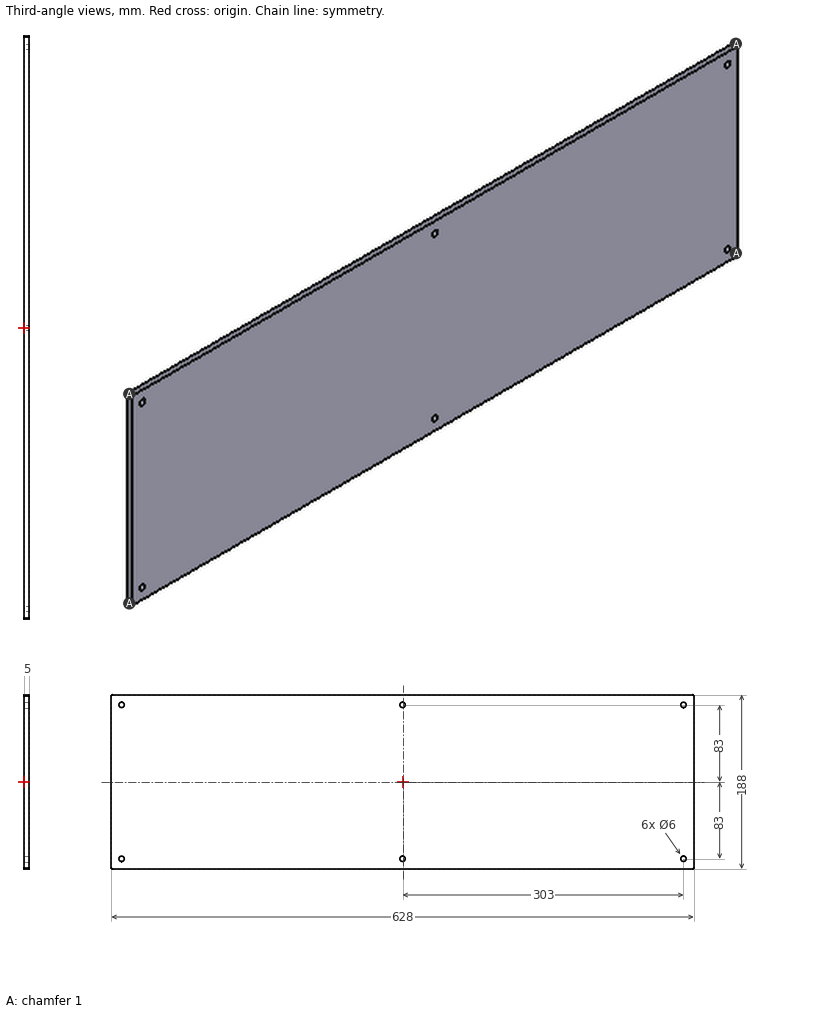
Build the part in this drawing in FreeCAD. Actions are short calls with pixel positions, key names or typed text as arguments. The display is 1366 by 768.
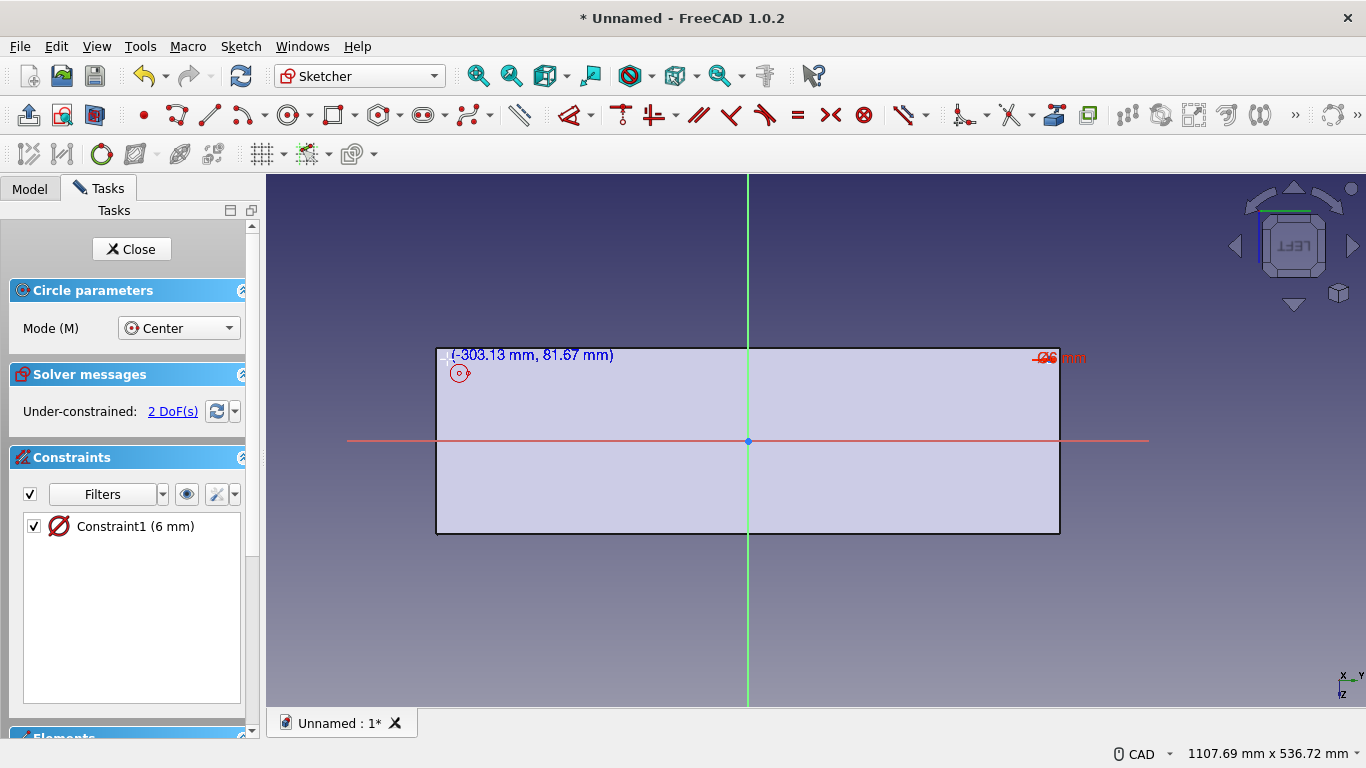
click(447, 359)
move(449, 357)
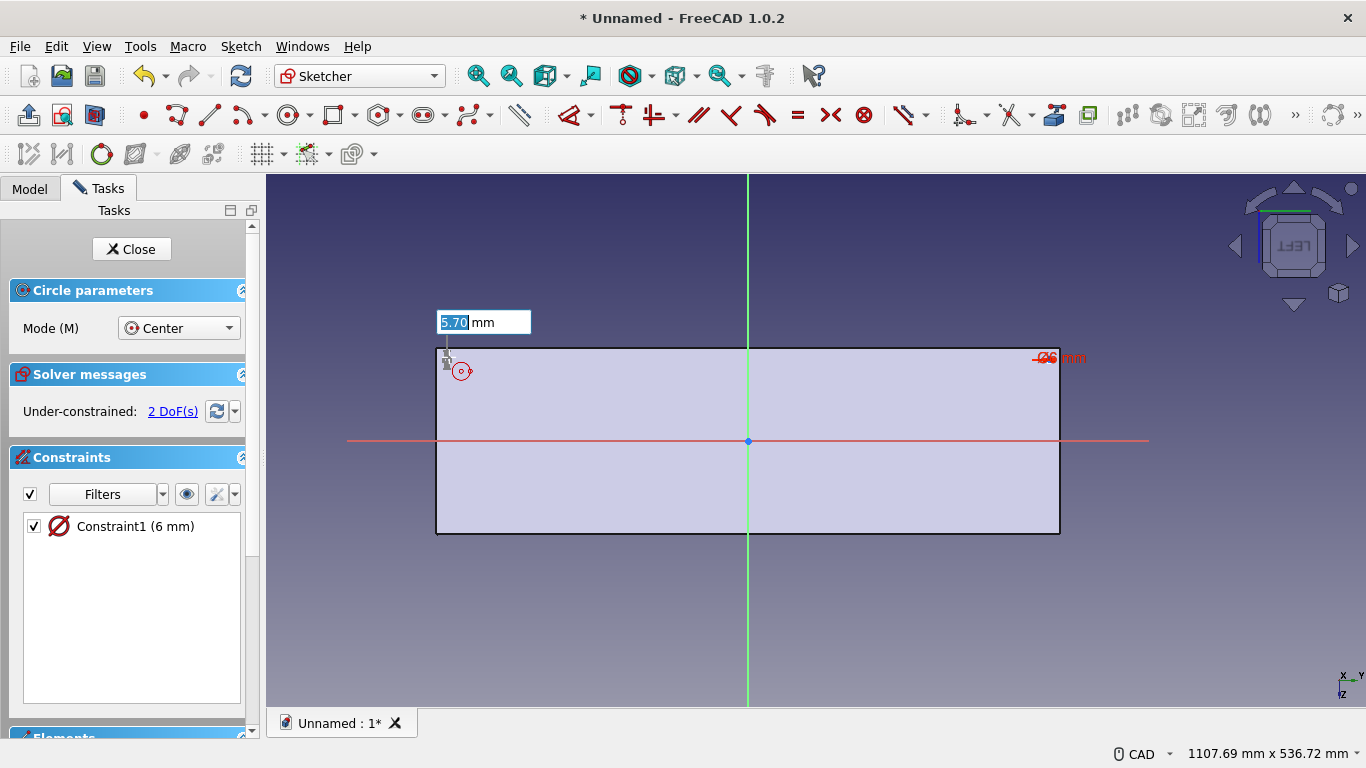
text(6)
key(Return)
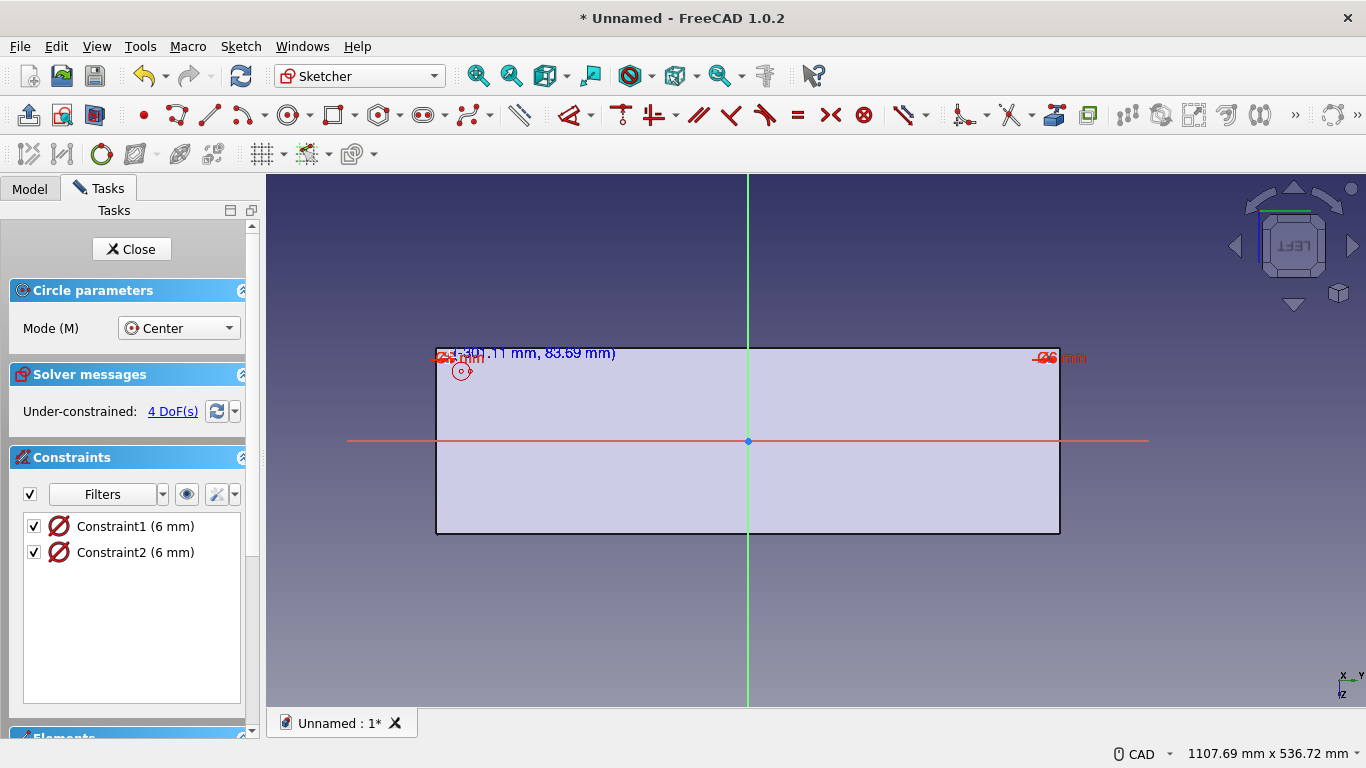
scroll(447, 524, up, 11)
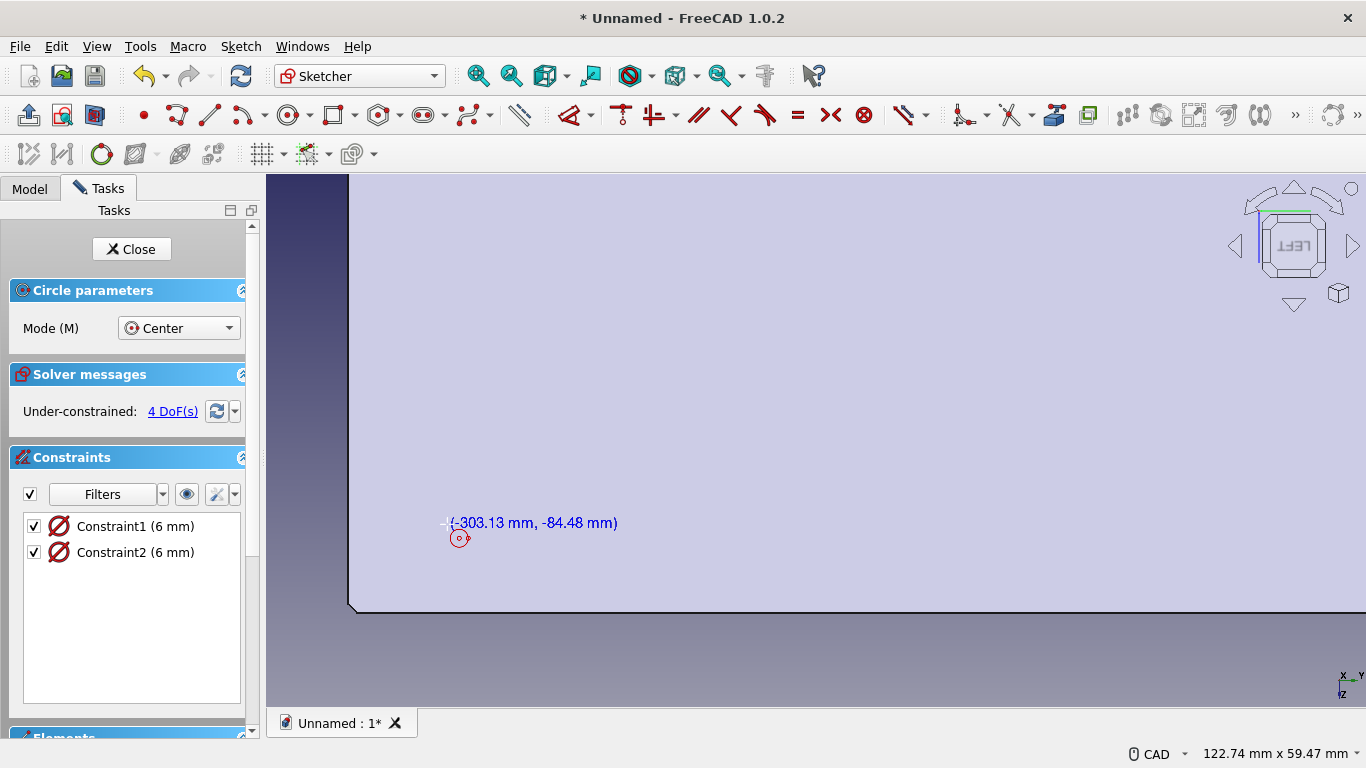
scroll(447, 524, down, 11)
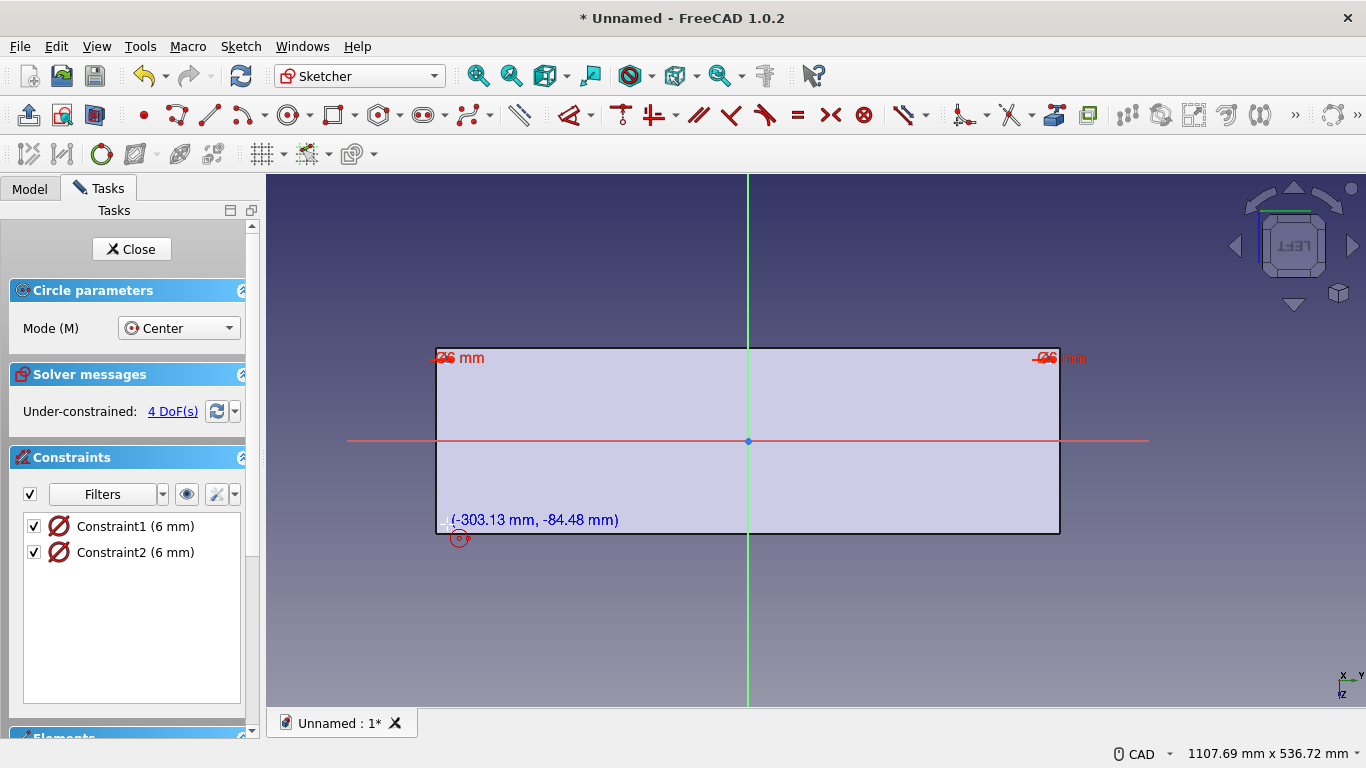
click(447, 524)
move(449, 521)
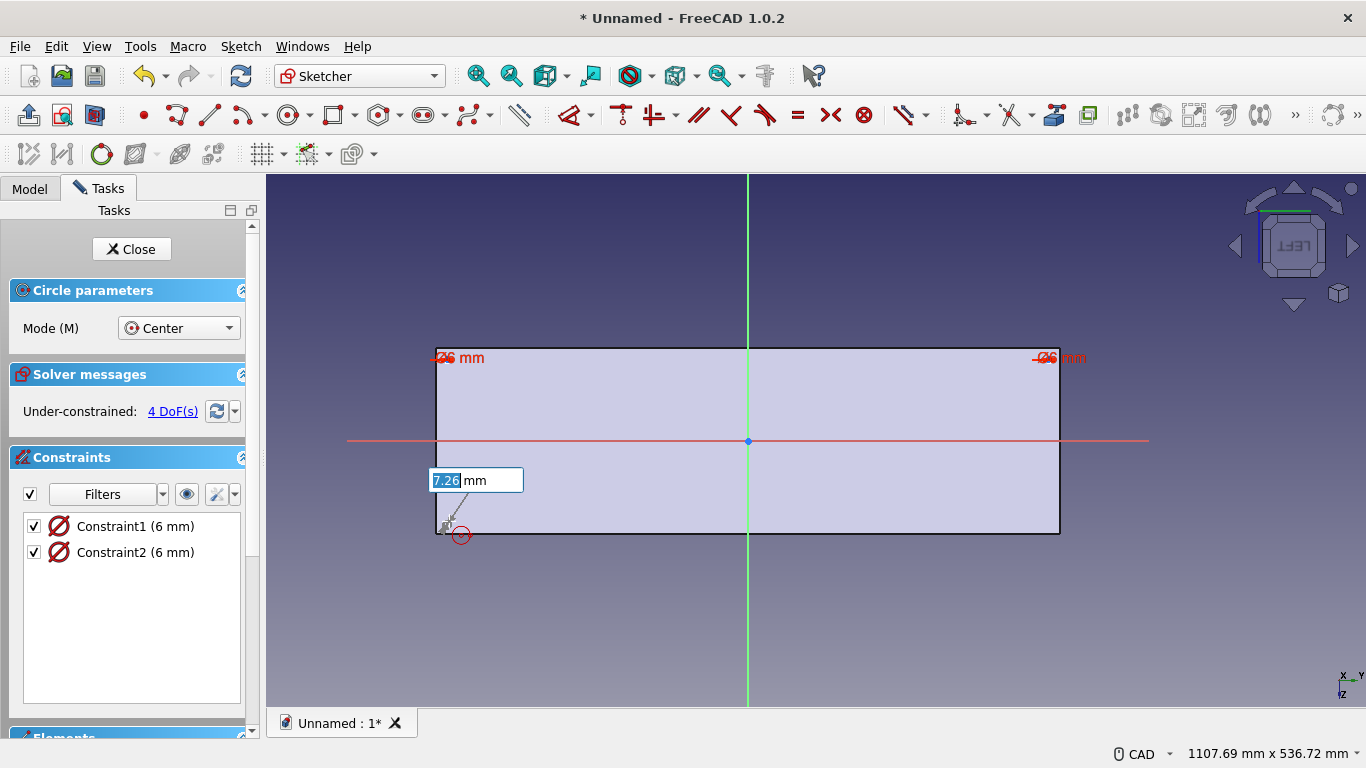
text(6)
key(Return)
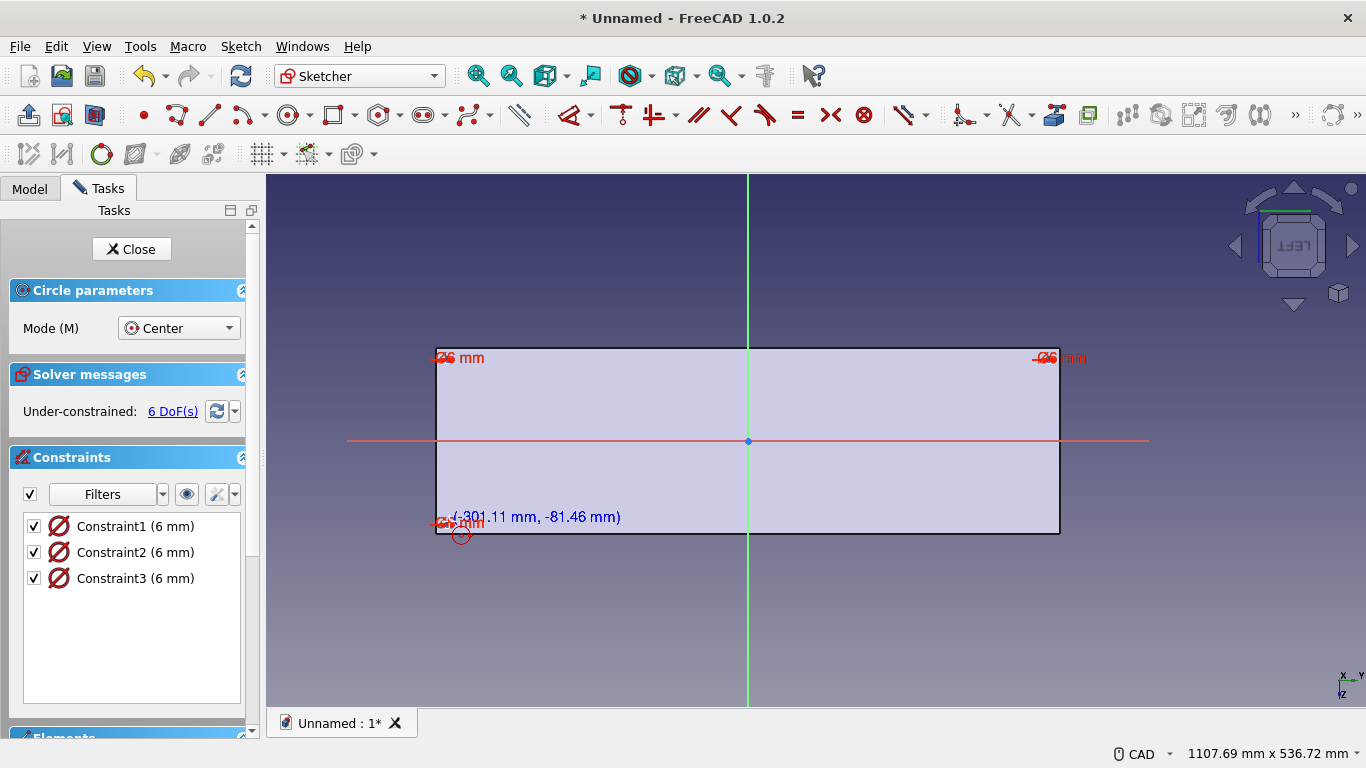
scroll(1049, 524, up, 11)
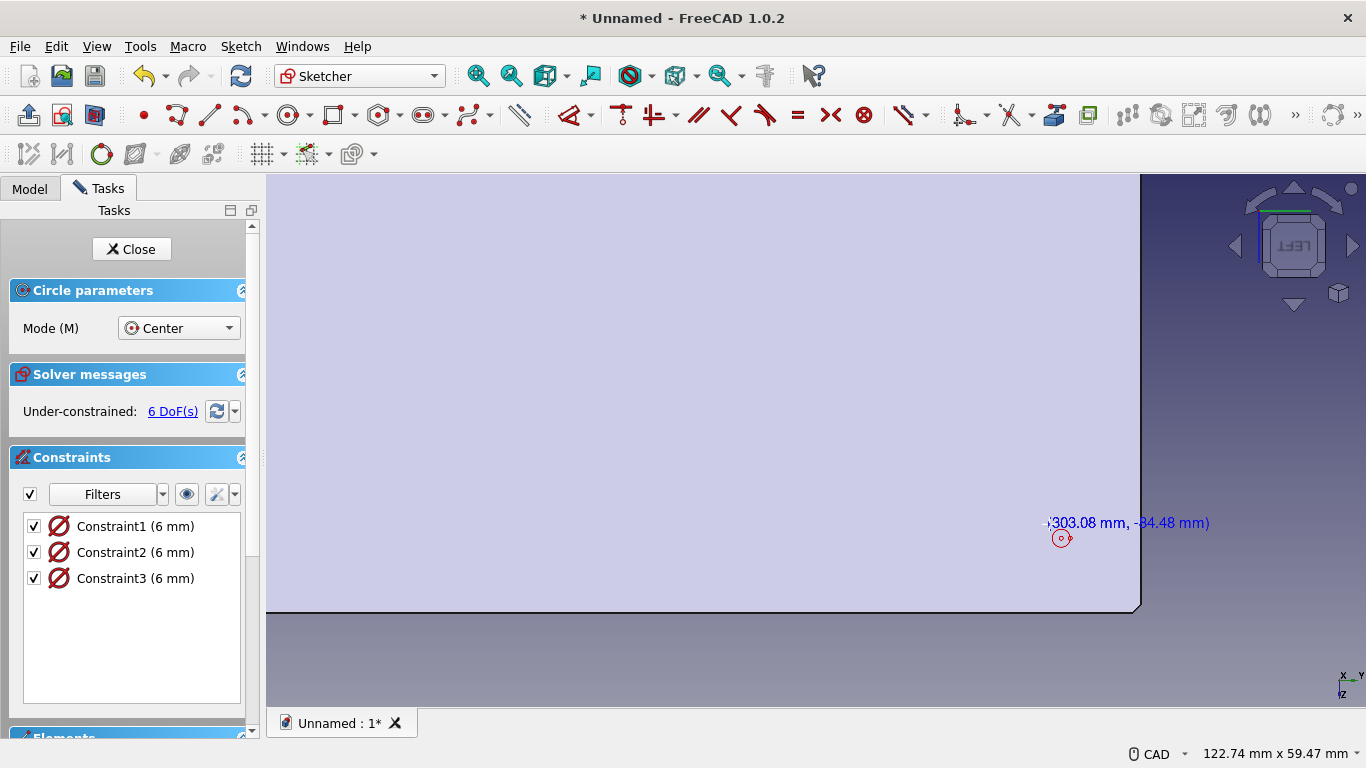
scroll(1049, 524, down, 11)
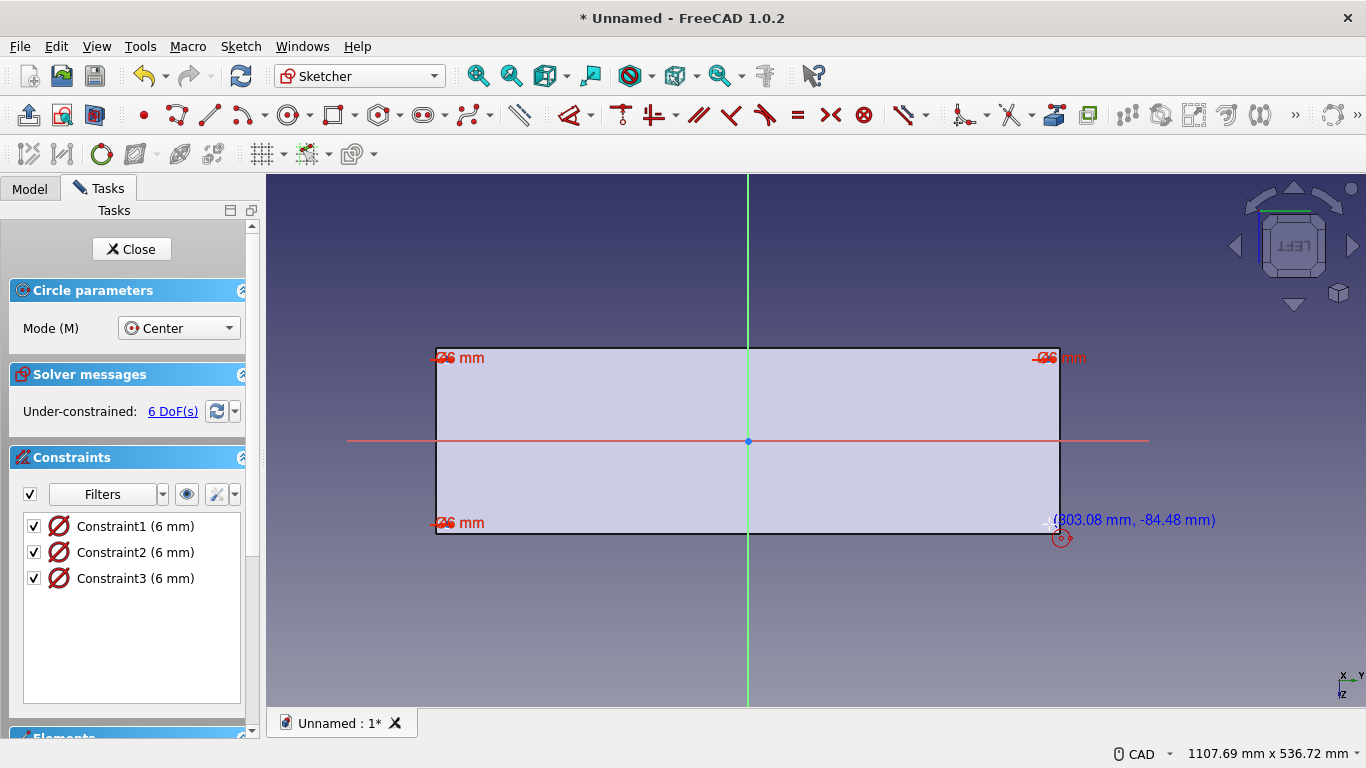
click(1049, 524)
move(1051, 521)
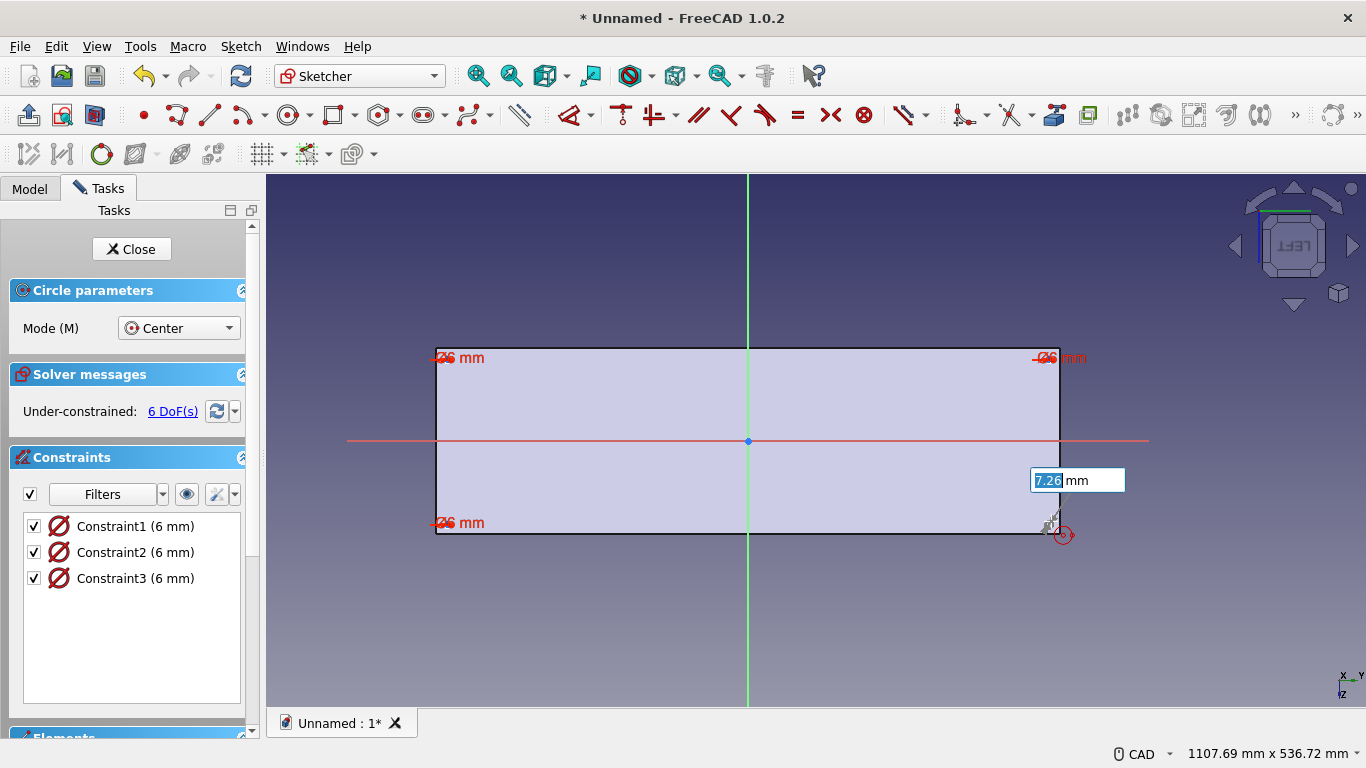
text(6)
key(Return)